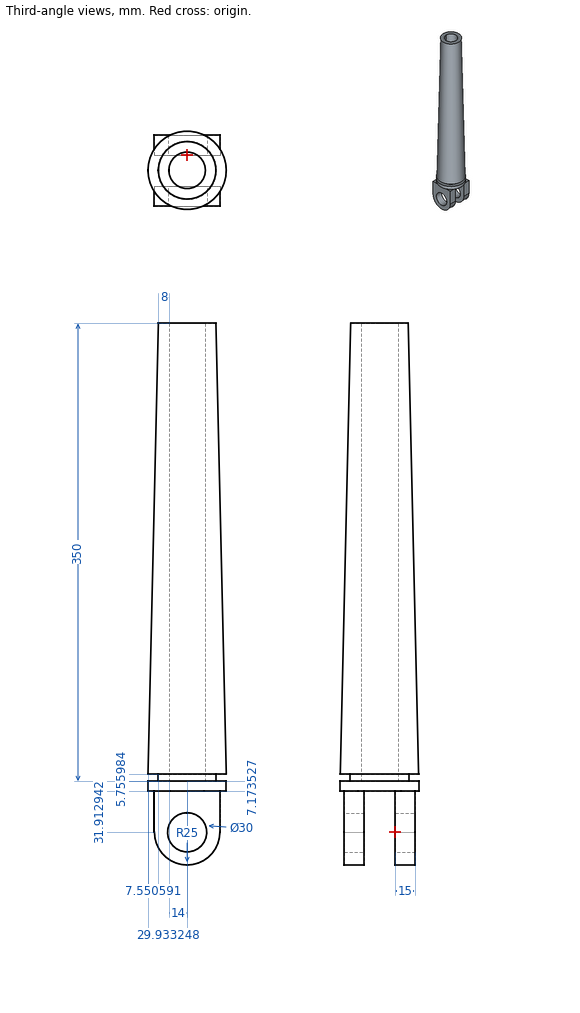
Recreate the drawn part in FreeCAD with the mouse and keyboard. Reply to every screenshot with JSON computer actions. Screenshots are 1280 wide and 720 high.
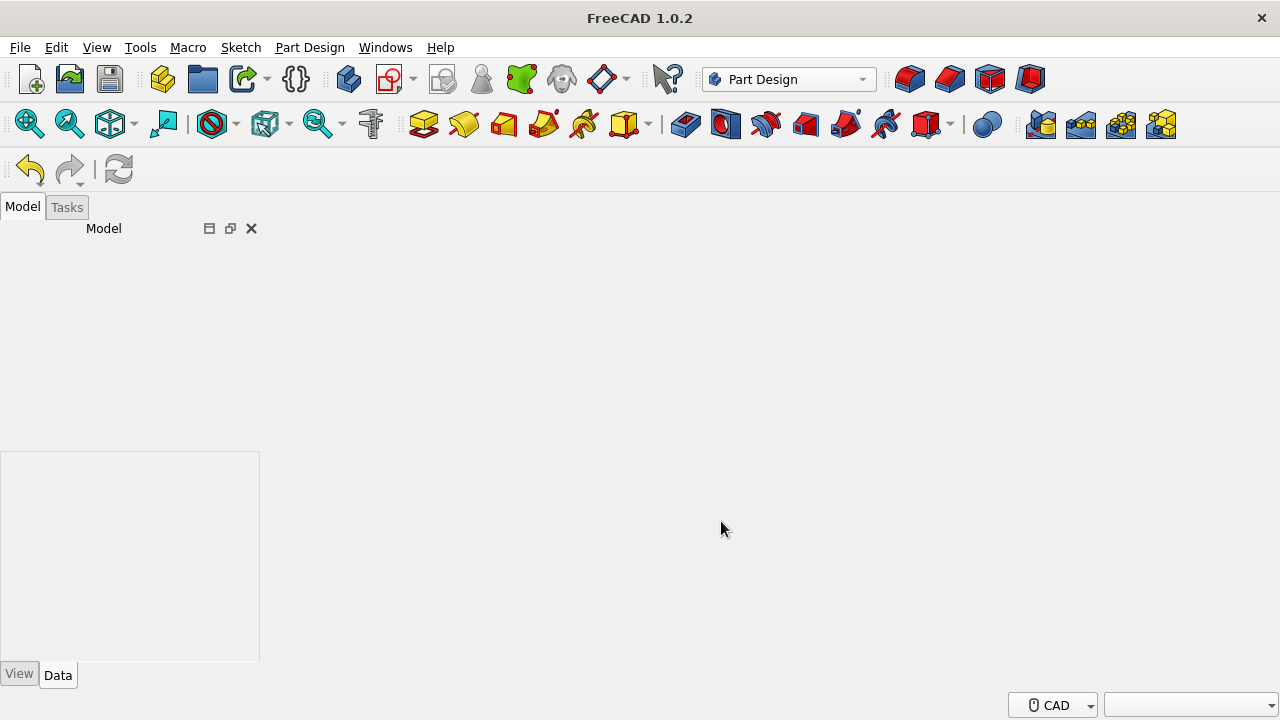
{"action": "left_click", "coordinate": [30, 80]}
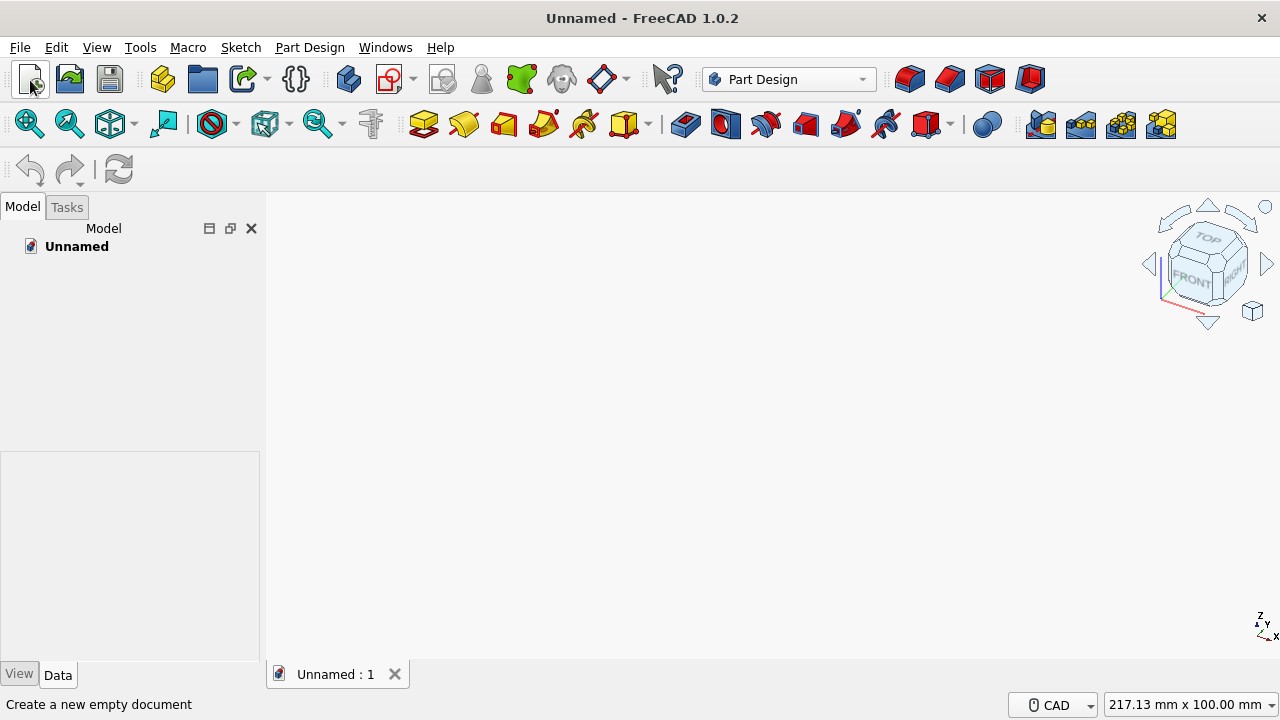
{"action": "left_click", "coordinate": [390, 80]}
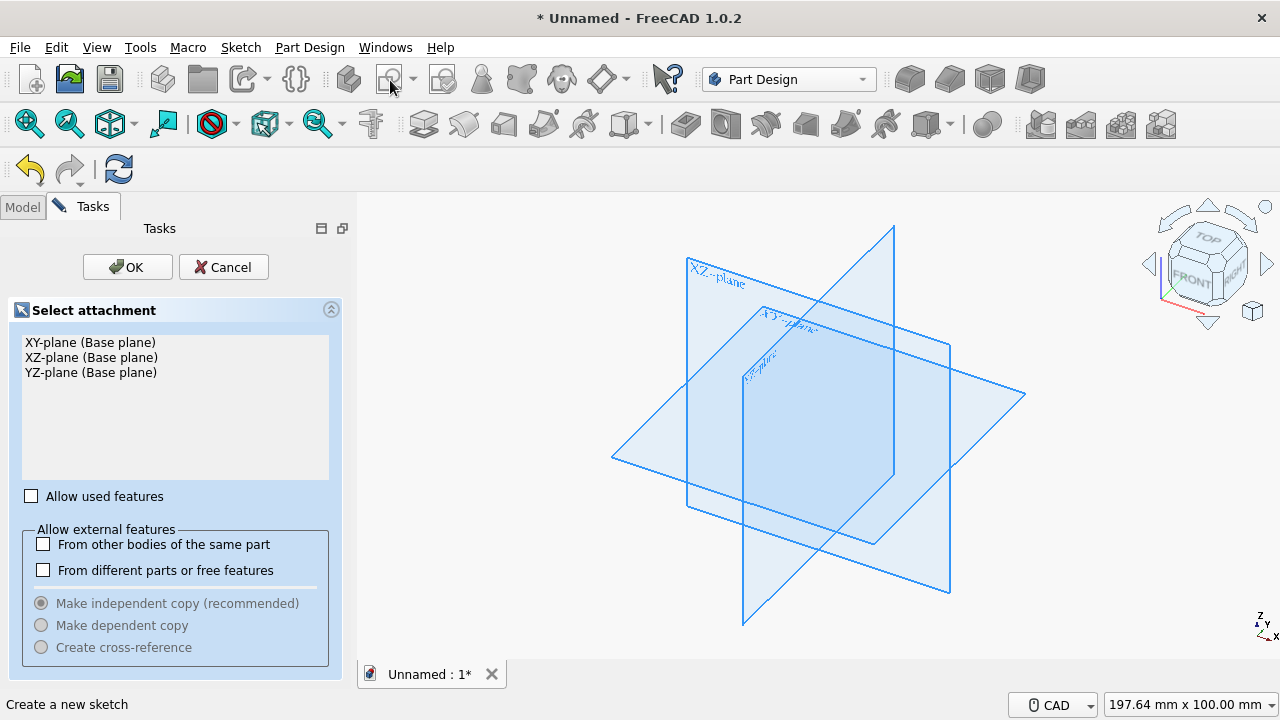
{"action": "left_click", "coordinate": [82, 358]}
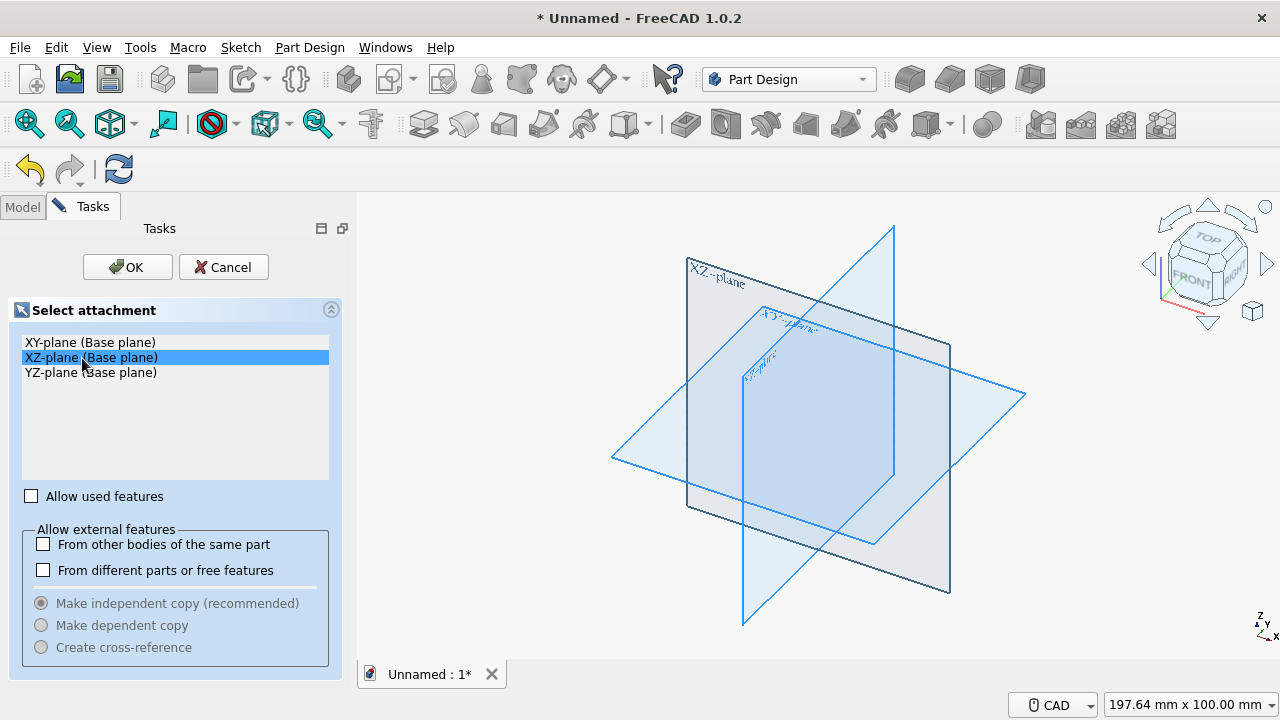
{"action": "left_click", "coordinate": [128, 267]}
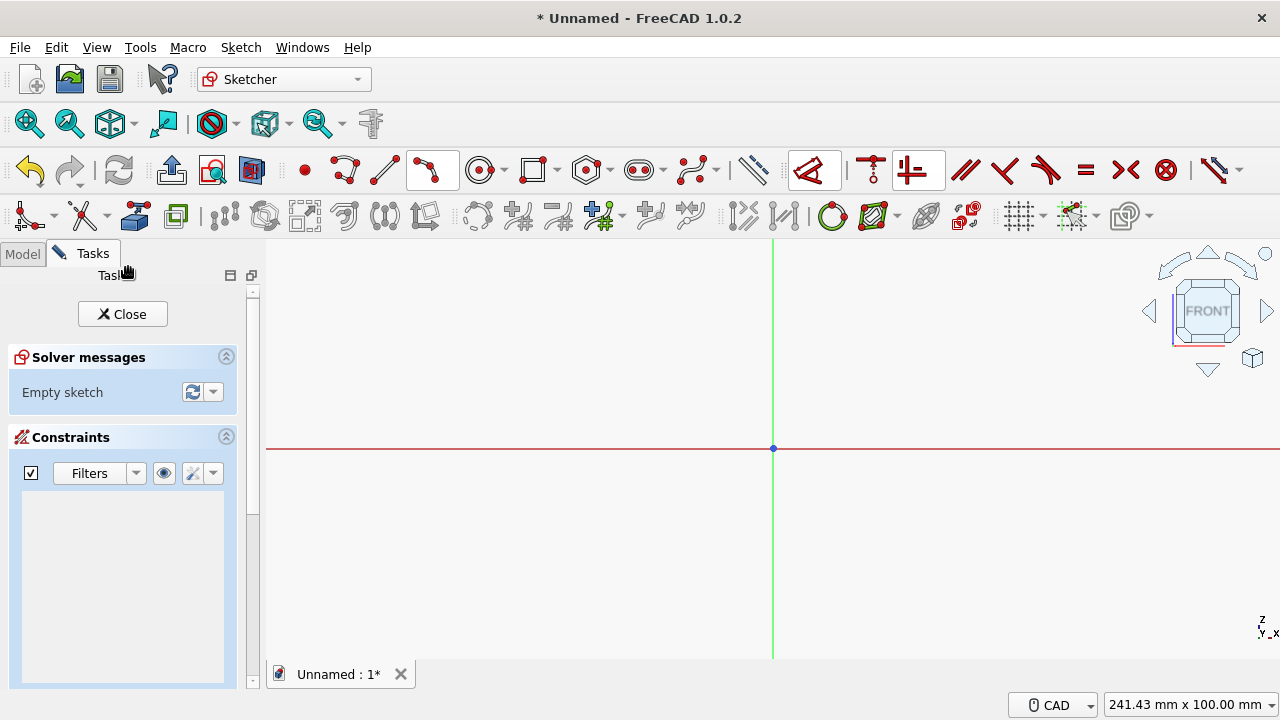
{"action": "left_click", "coordinate": [346, 170]}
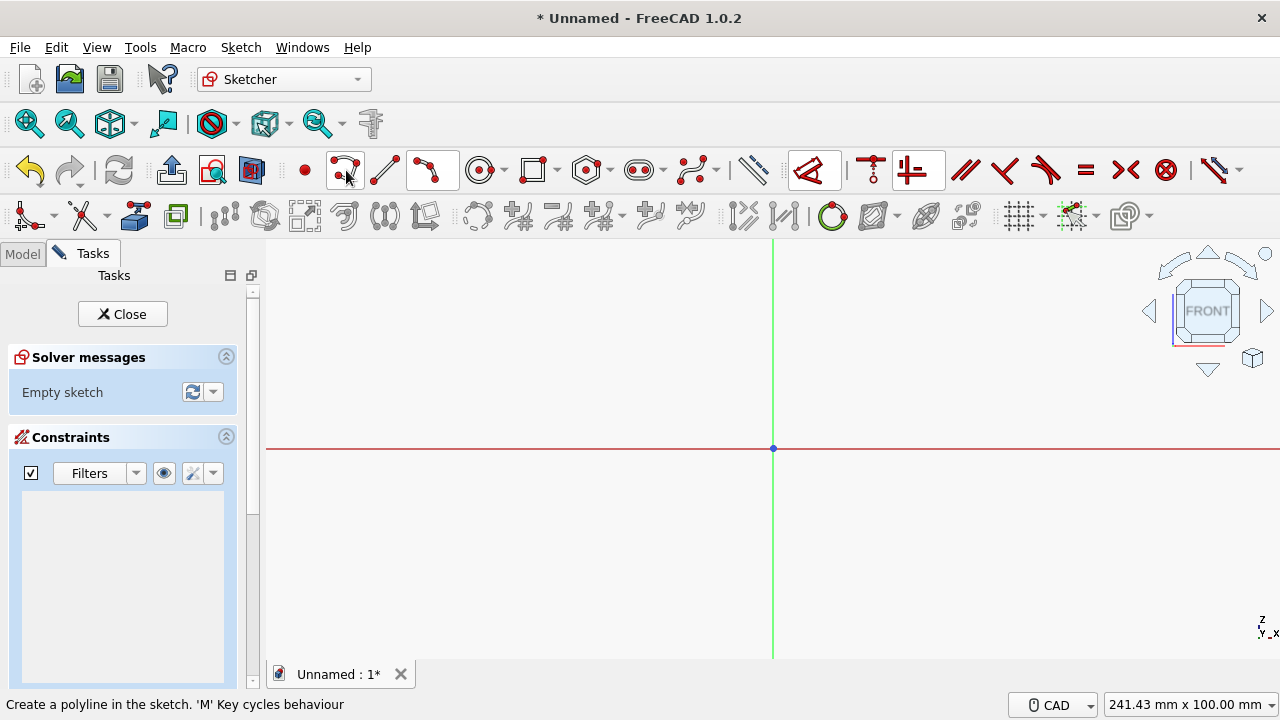
{"action": "left_click", "coordinate": [668, 449]}
{"action": "left_click", "coordinate": [668, 315]}
{"action": "left_click", "coordinate": [878, 315]}
{"action": "left_click", "coordinate": [878, 449]}
{"action": "right_click", "coordinate": [878, 449]}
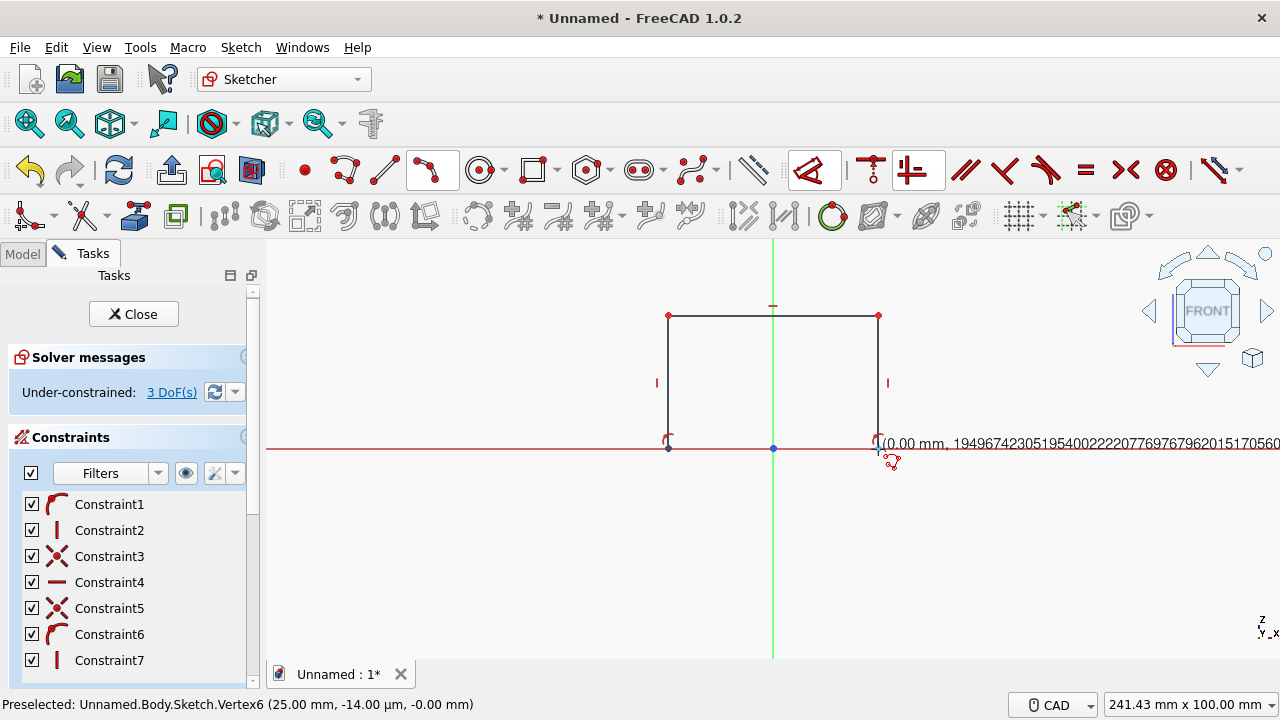
{"action": "left_click", "coordinate": [426, 170]}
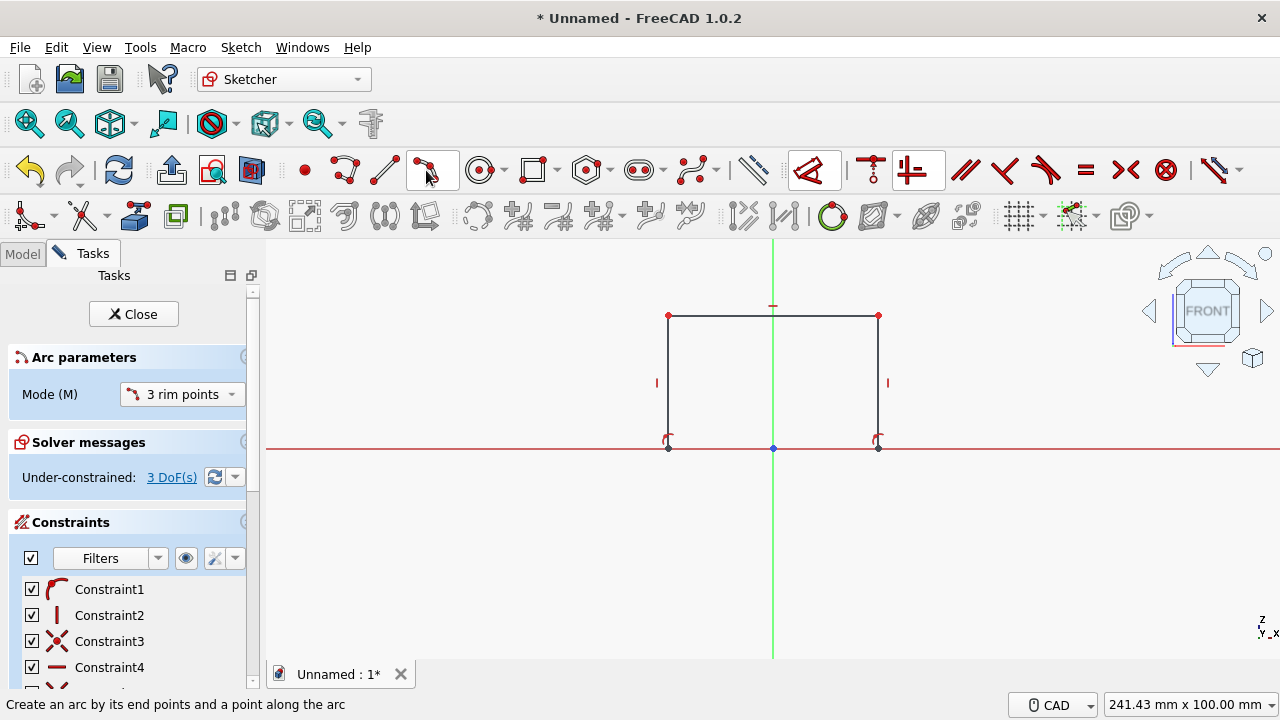
{"action": "left_click", "coordinate": [878, 449]}
{"action": "left_click", "coordinate": [668, 449]}
{"action": "left_click", "coordinate": [741, 549]}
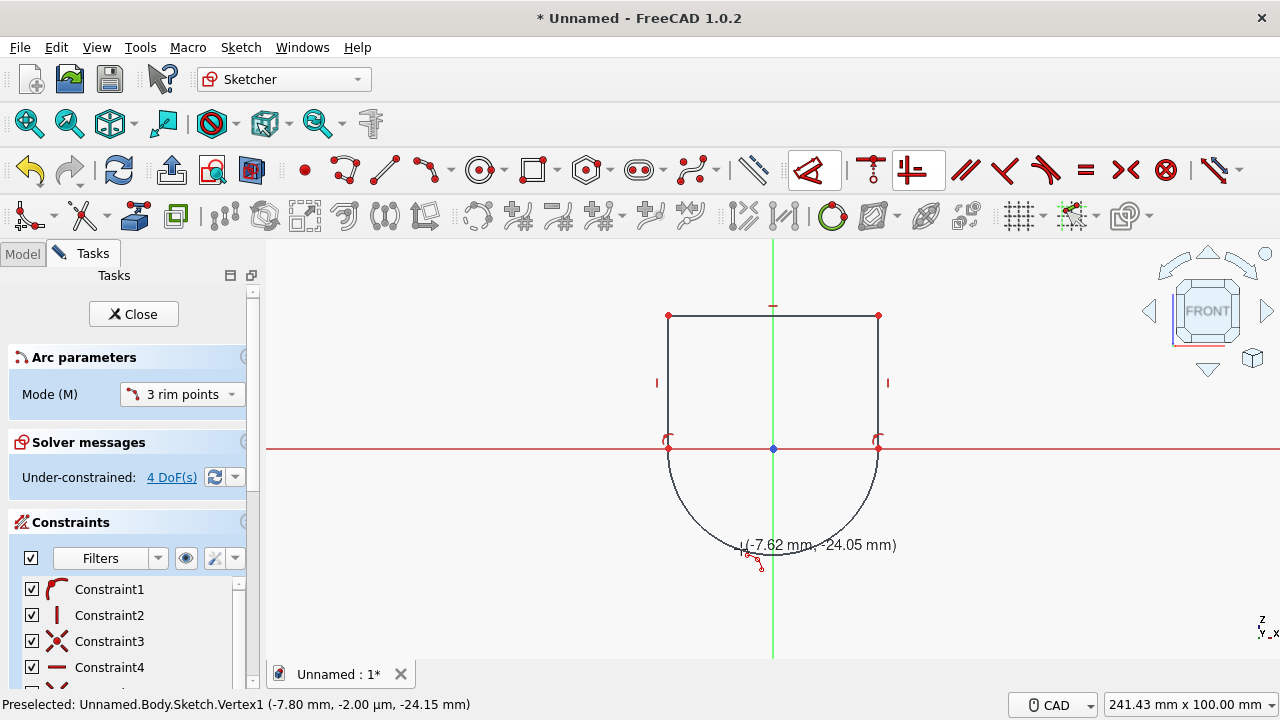
{"action": "left_click", "coordinate": [480, 170]}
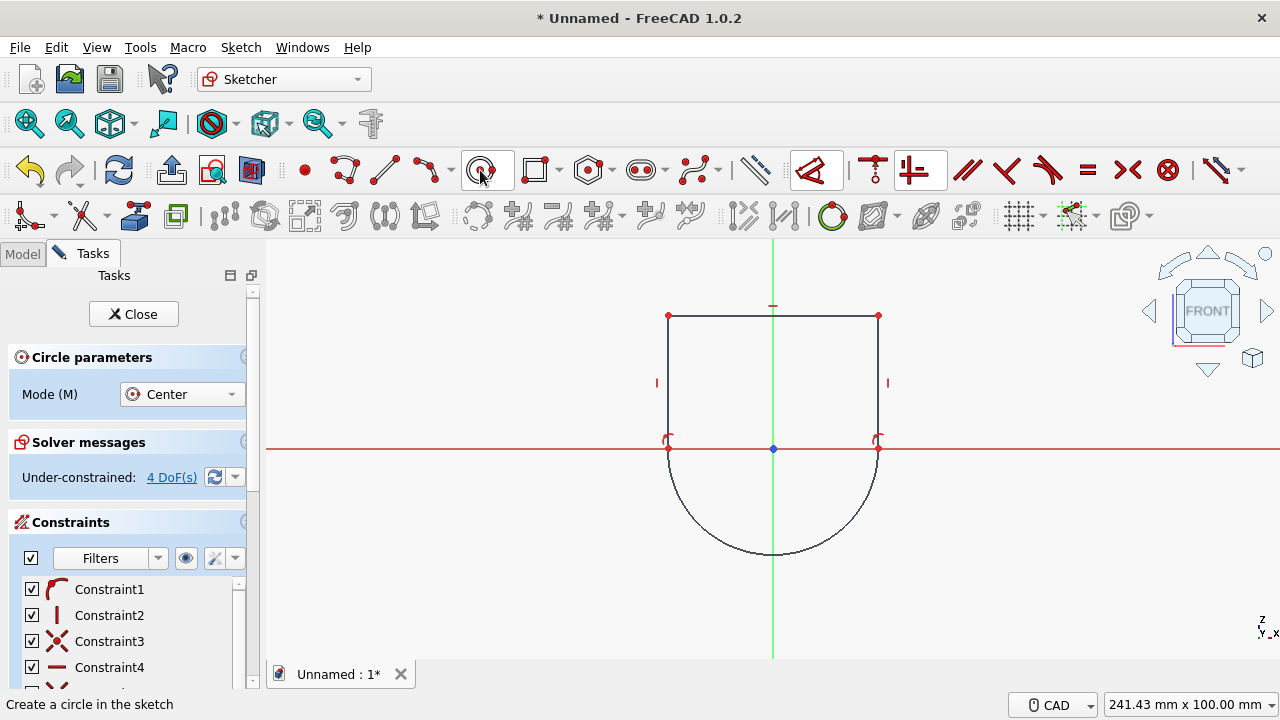
{"action": "left_click", "coordinate": [773, 449]}
{"action": "mouse_move", "coordinate": [818, 404]}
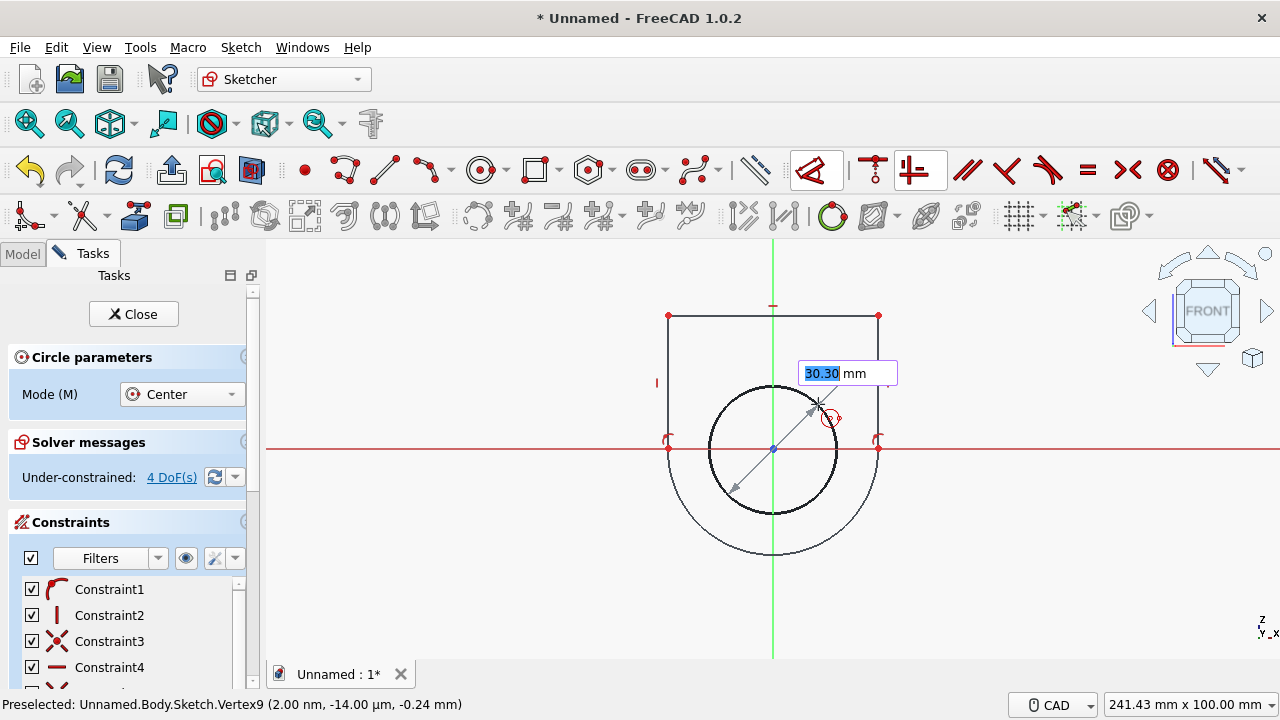
{"action": "type", "text": "30"}
{"action": "key", "text": "Return"}
{"action": "key", "text": "Escape"}